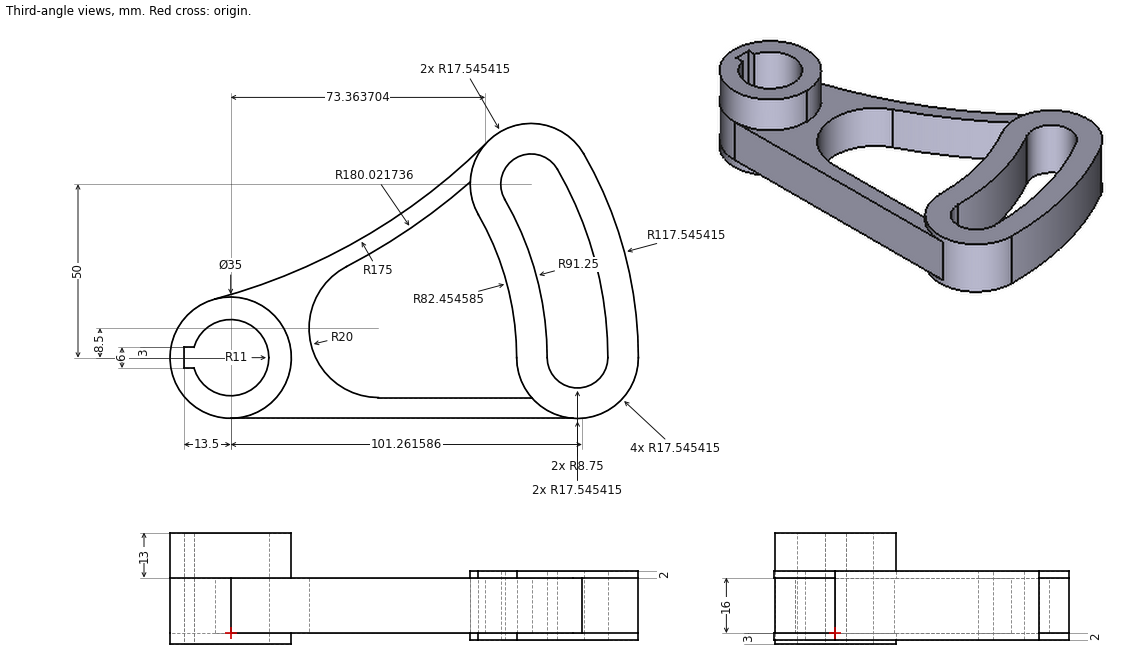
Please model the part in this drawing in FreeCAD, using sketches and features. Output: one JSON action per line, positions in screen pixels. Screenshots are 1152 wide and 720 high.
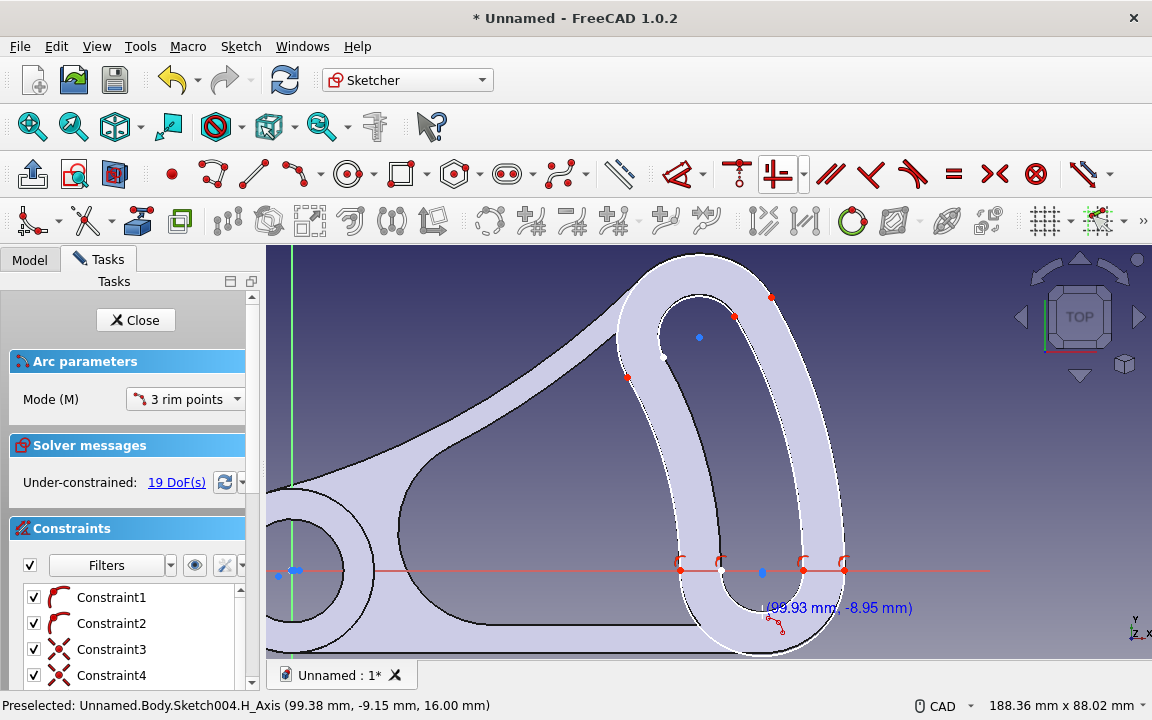
{"action": "left_click", "coordinate": [721, 571]}
{"action": "left_click", "coordinate": [664, 357]}
{"action": "left_click", "coordinate": [707, 460]}
{"action": "key", "text": "Escape"}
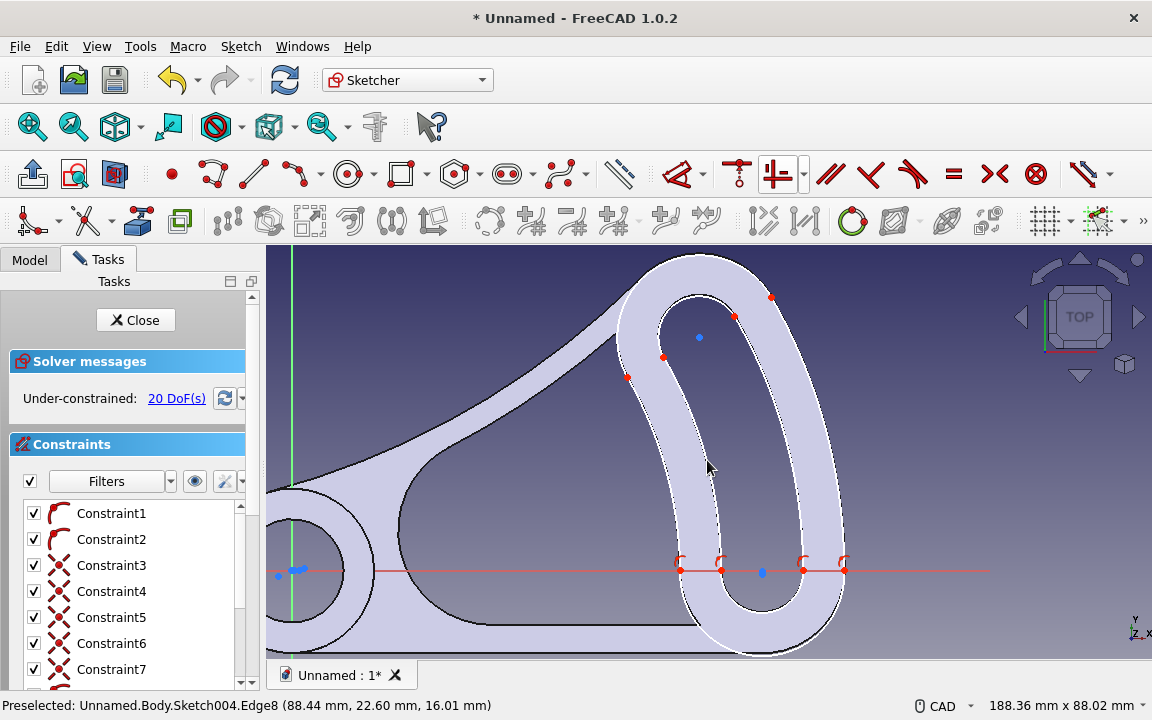
{"action": "left_click", "coordinate": [695, 621]}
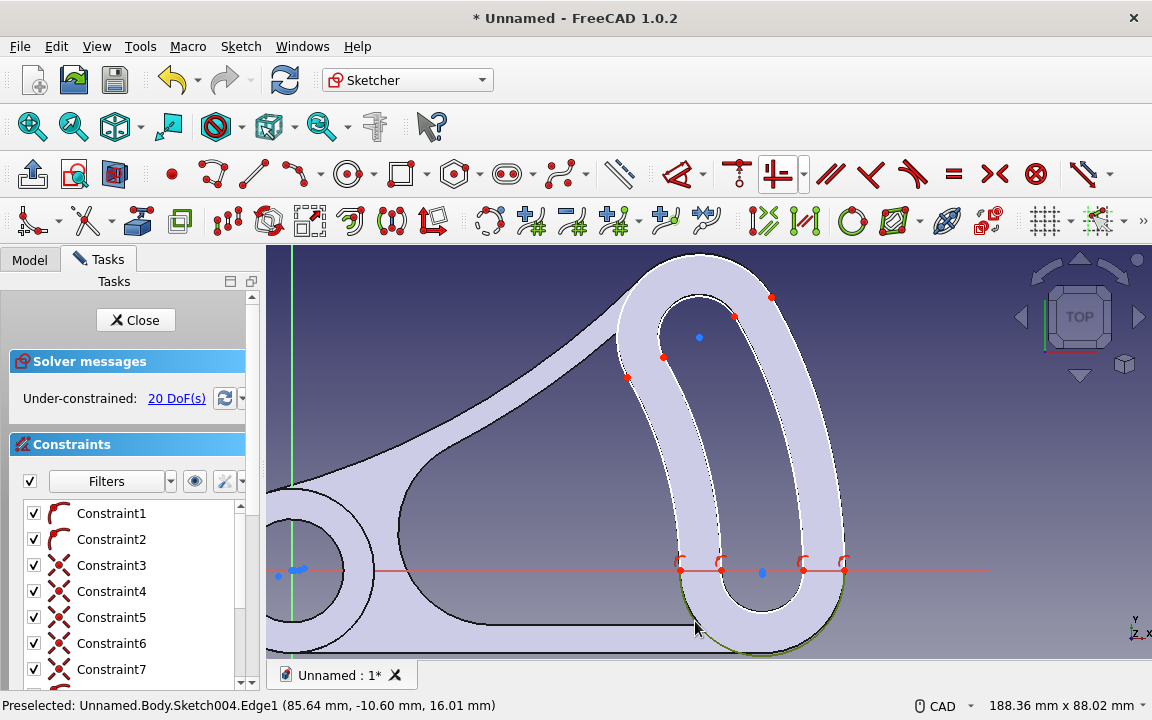
{"action": "left_click", "coordinate": [838, 485]}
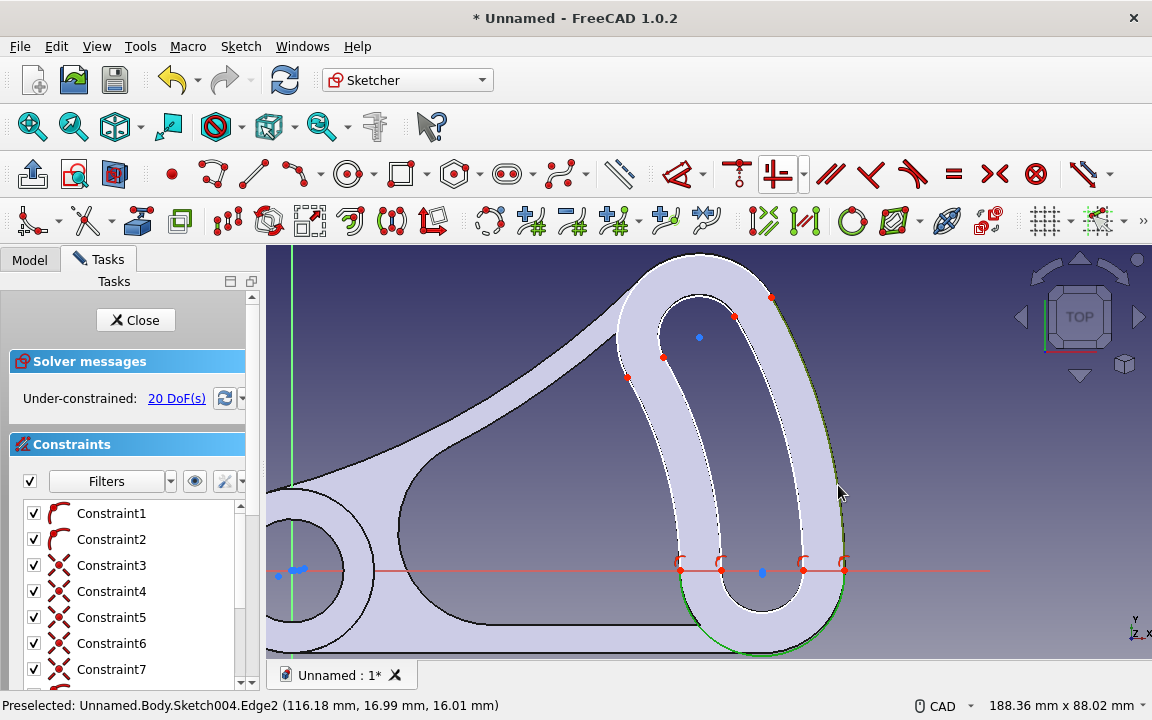
{"action": "left_click", "coordinate": [913, 174]}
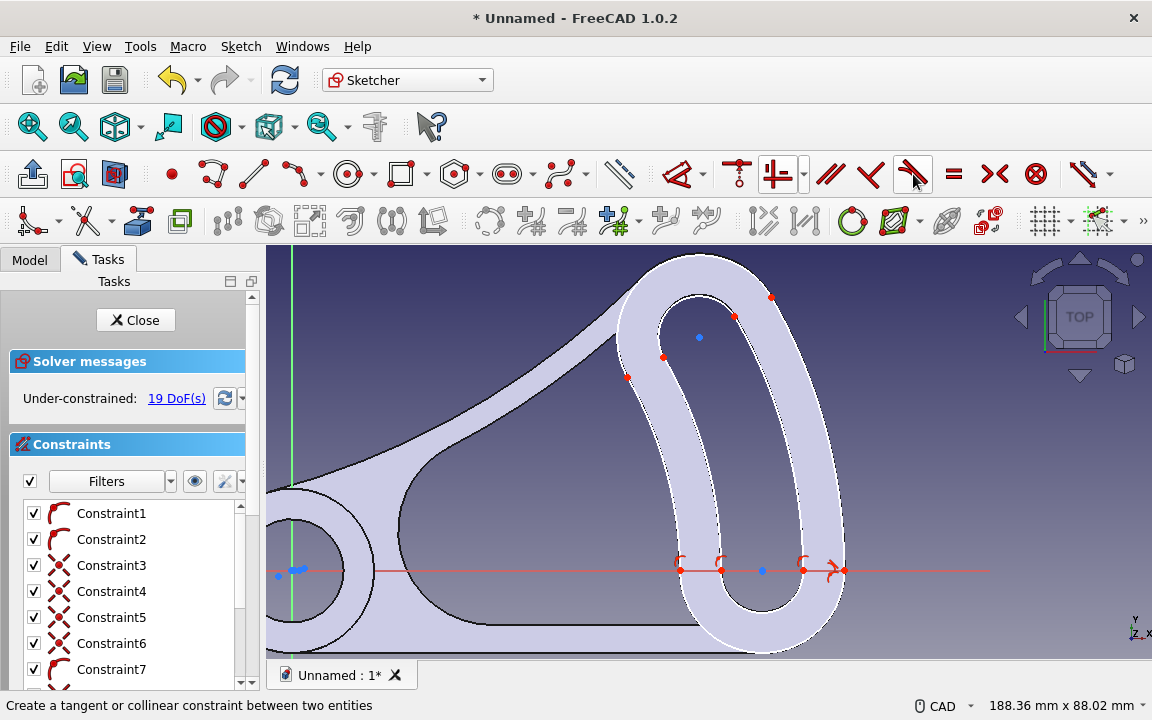
{"action": "left_click", "coordinate": [838, 485]}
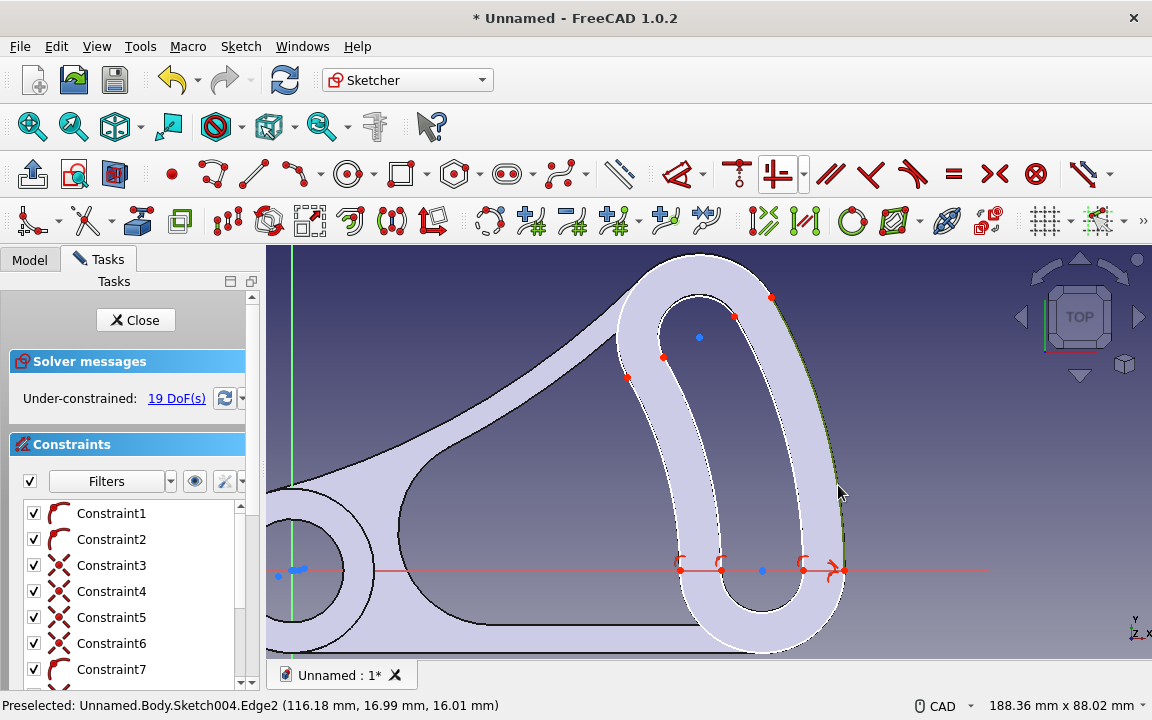
{"action": "left_click", "coordinate": [625, 303]}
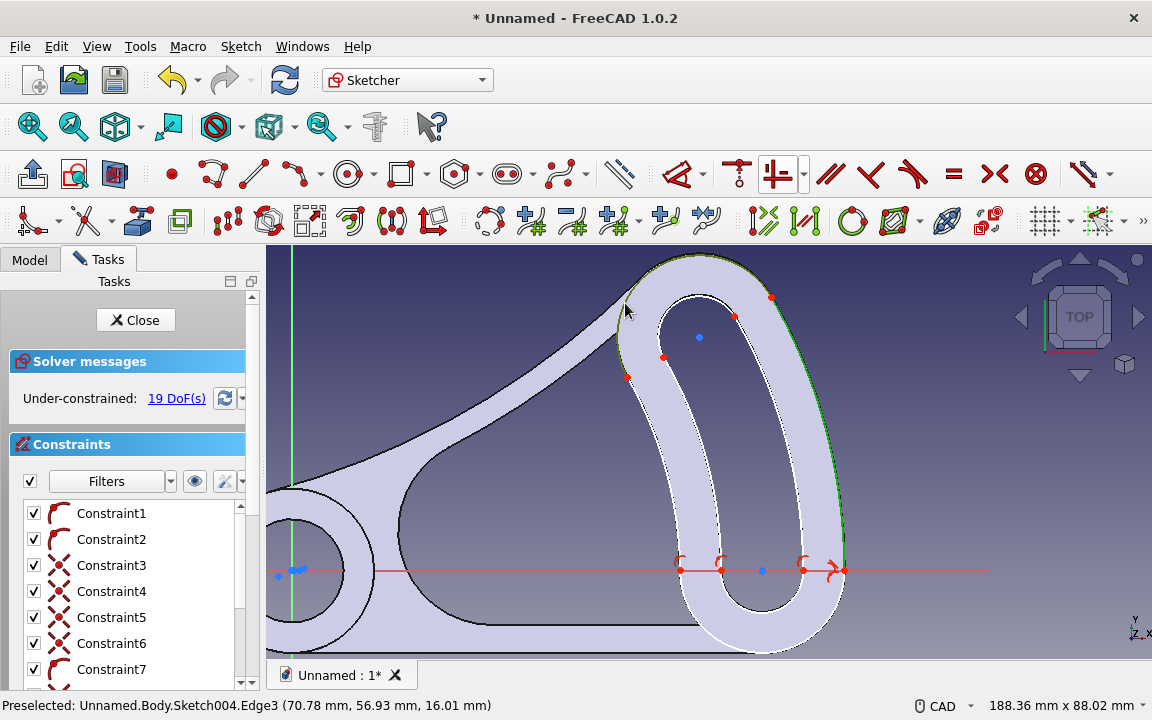
{"action": "left_click", "coordinate": [913, 174]}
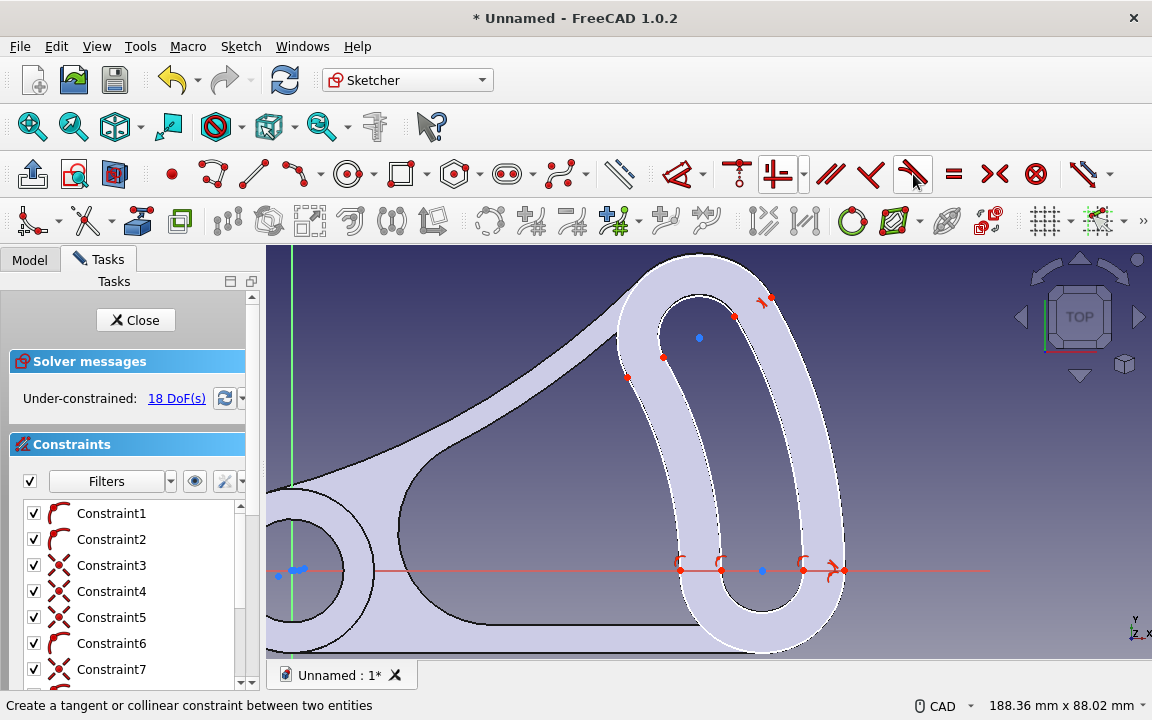
{"action": "left_click", "coordinate": [625, 303]}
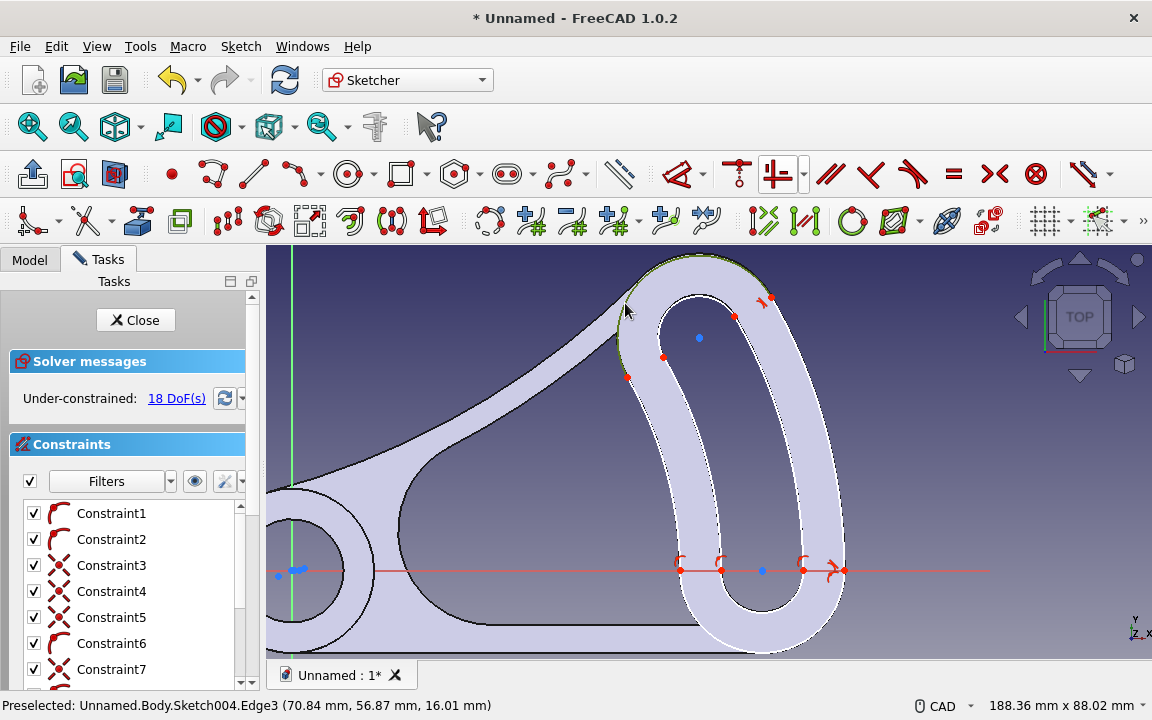
{"action": "left_click", "coordinate": [675, 510]}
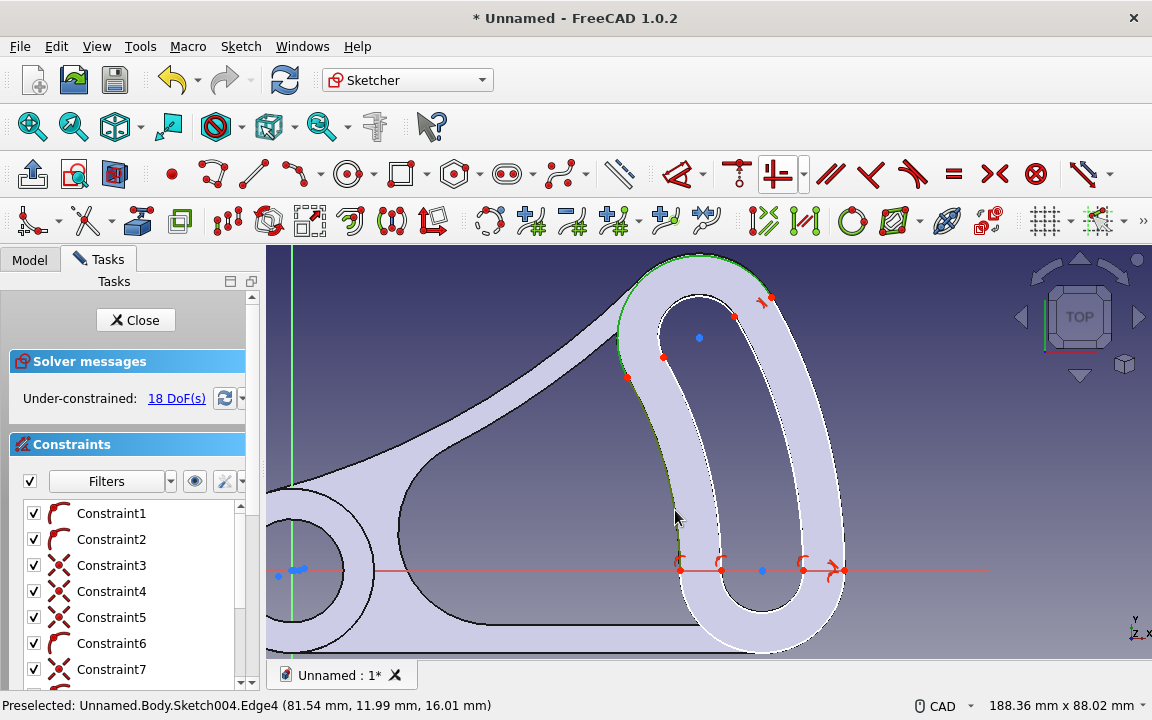
{"action": "left_click", "coordinate": [913, 174]}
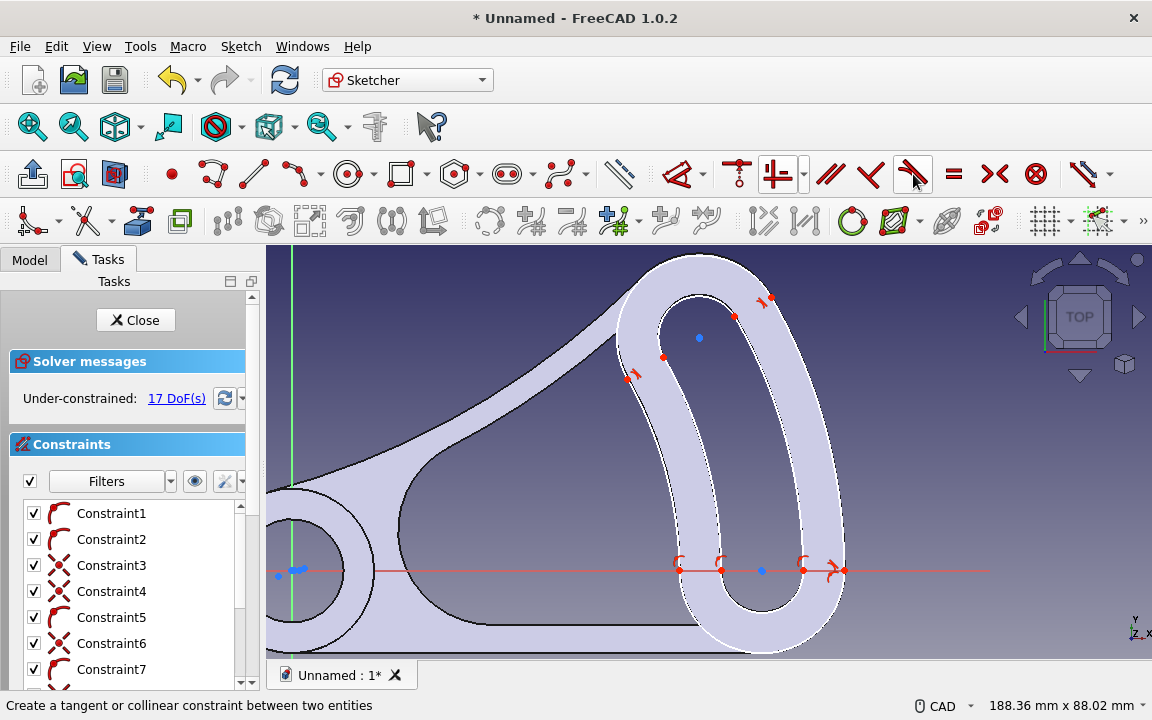
{"action": "left_click", "coordinate": [703, 297]}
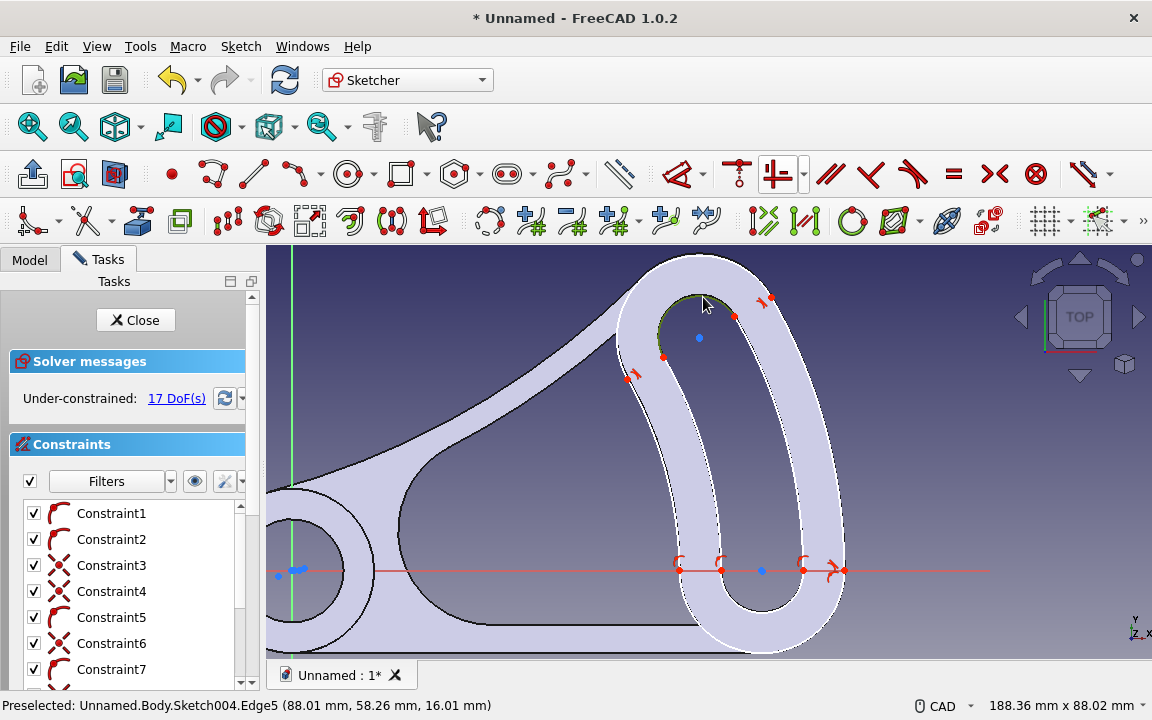
{"action": "left_click", "coordinate": [797, 491]}